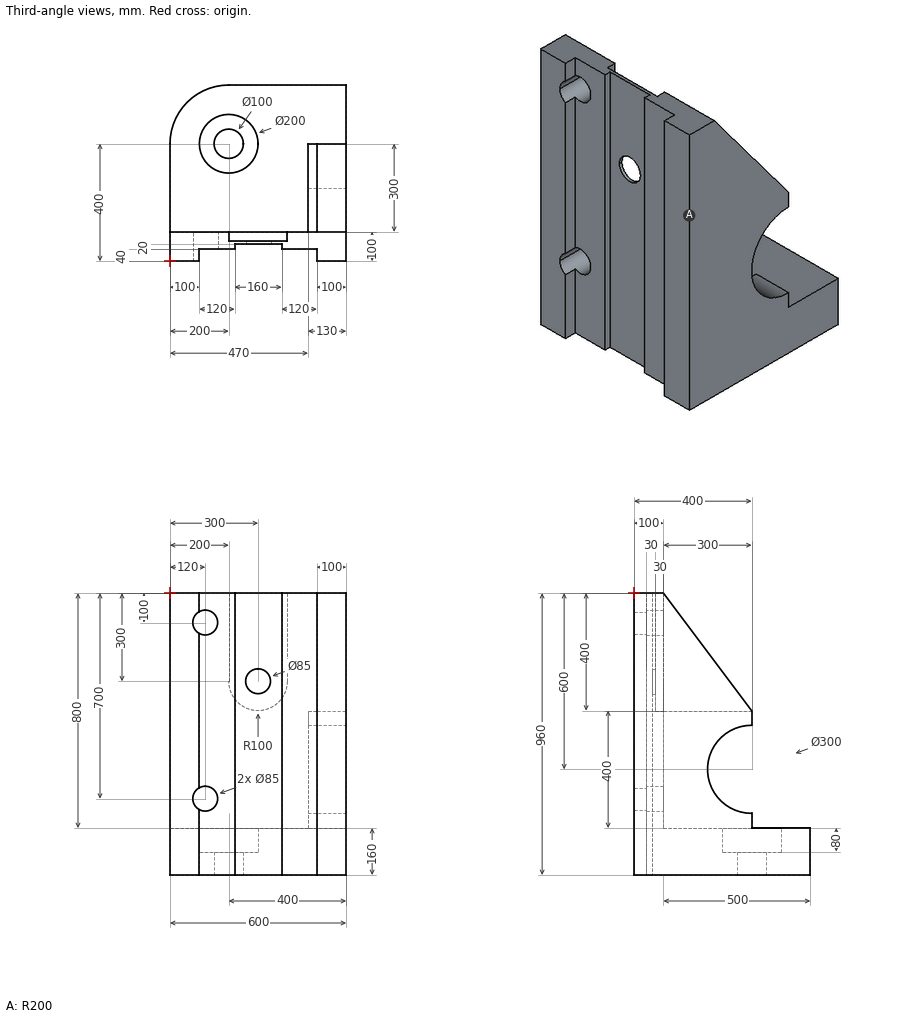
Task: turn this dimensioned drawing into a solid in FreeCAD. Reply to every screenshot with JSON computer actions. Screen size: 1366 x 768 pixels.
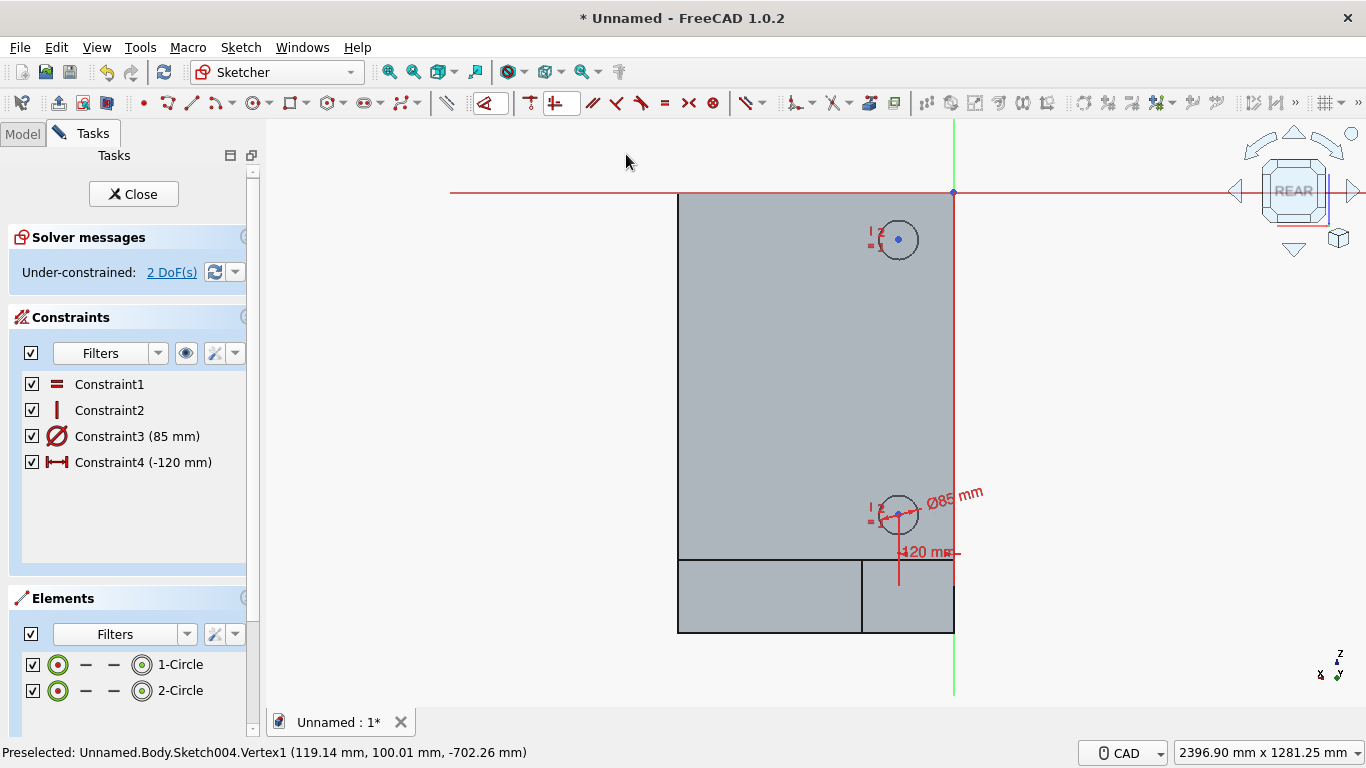
{"action": "left_click", "coordinate": [899, 515]}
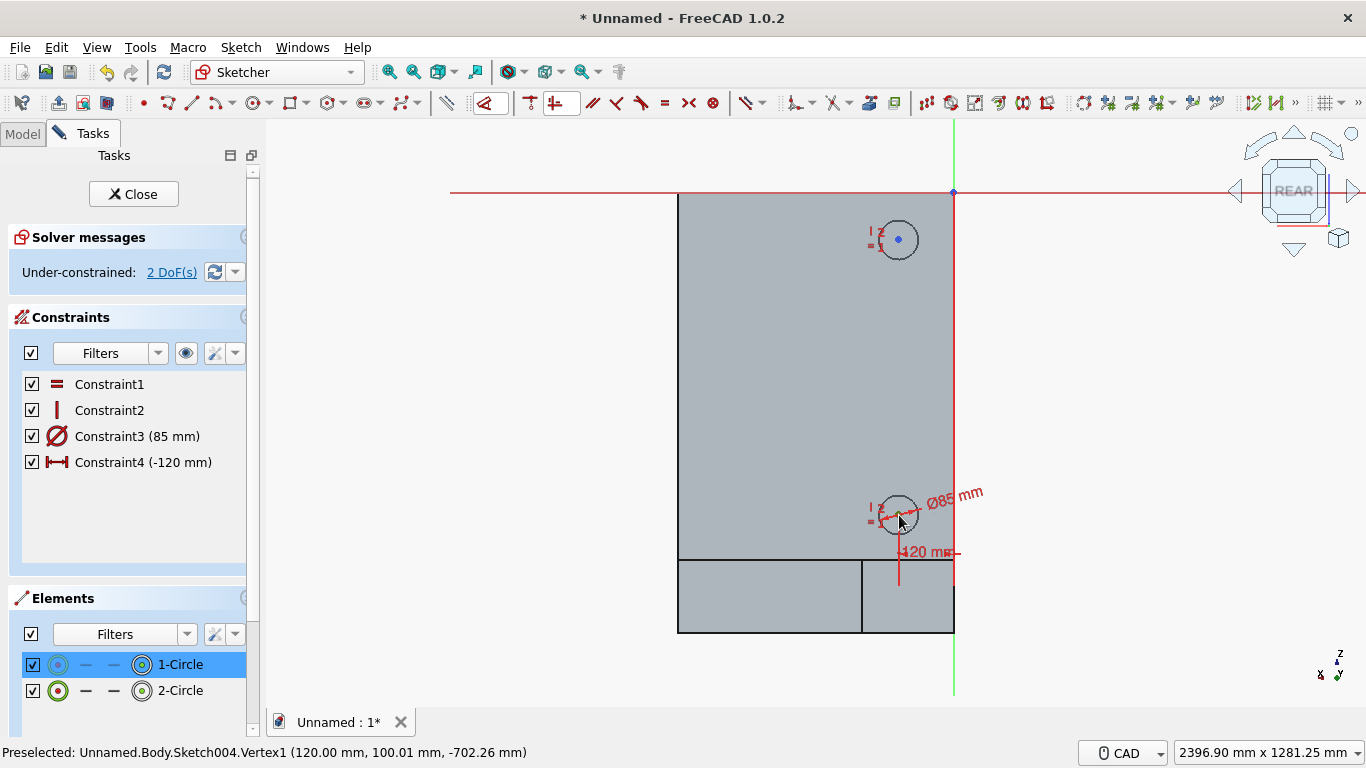
{"action": "left_click", "coordinate": [502, 104]}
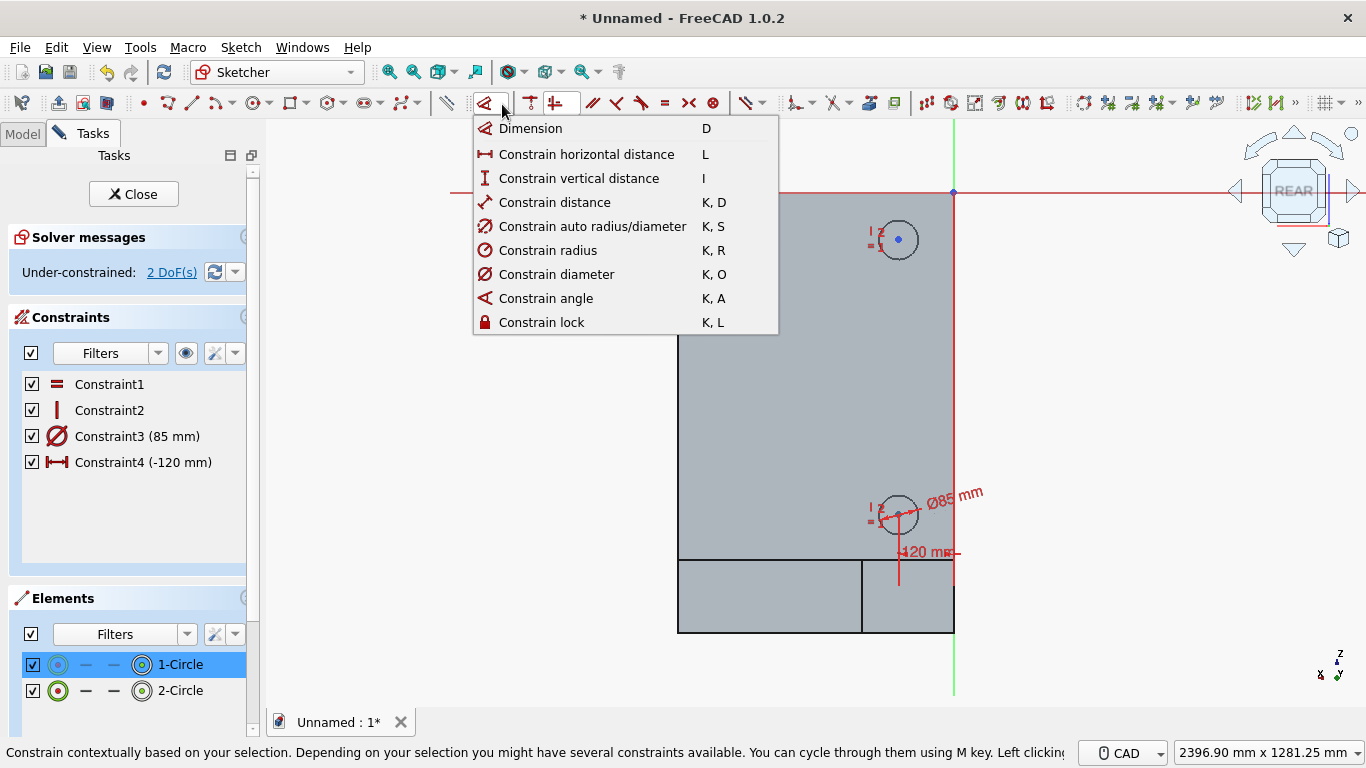
{"action": "left_click", "coordinate": [626, 178]}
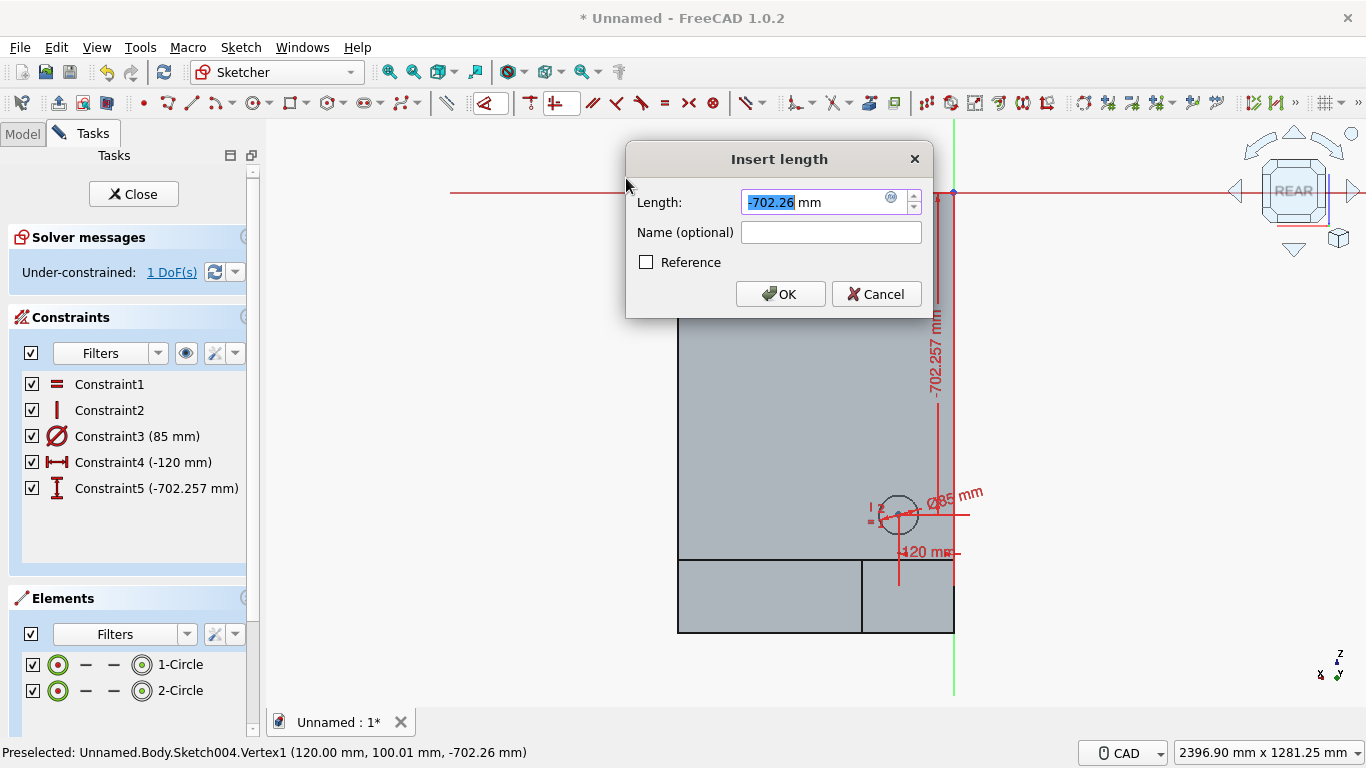
{"action": "type", "text": "-700"}
{"action": "key", "text": "Return"}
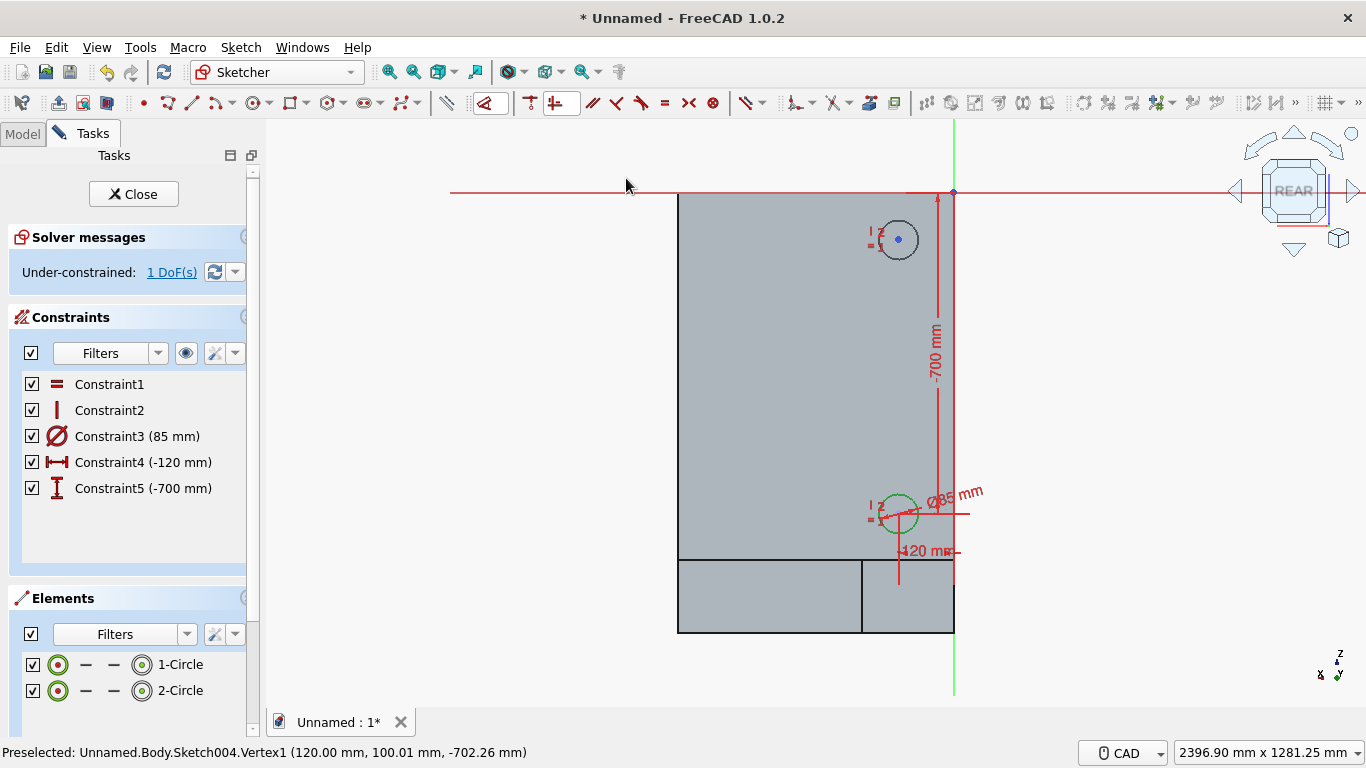
{"action": "left_click", "coordinate": [899, 240]}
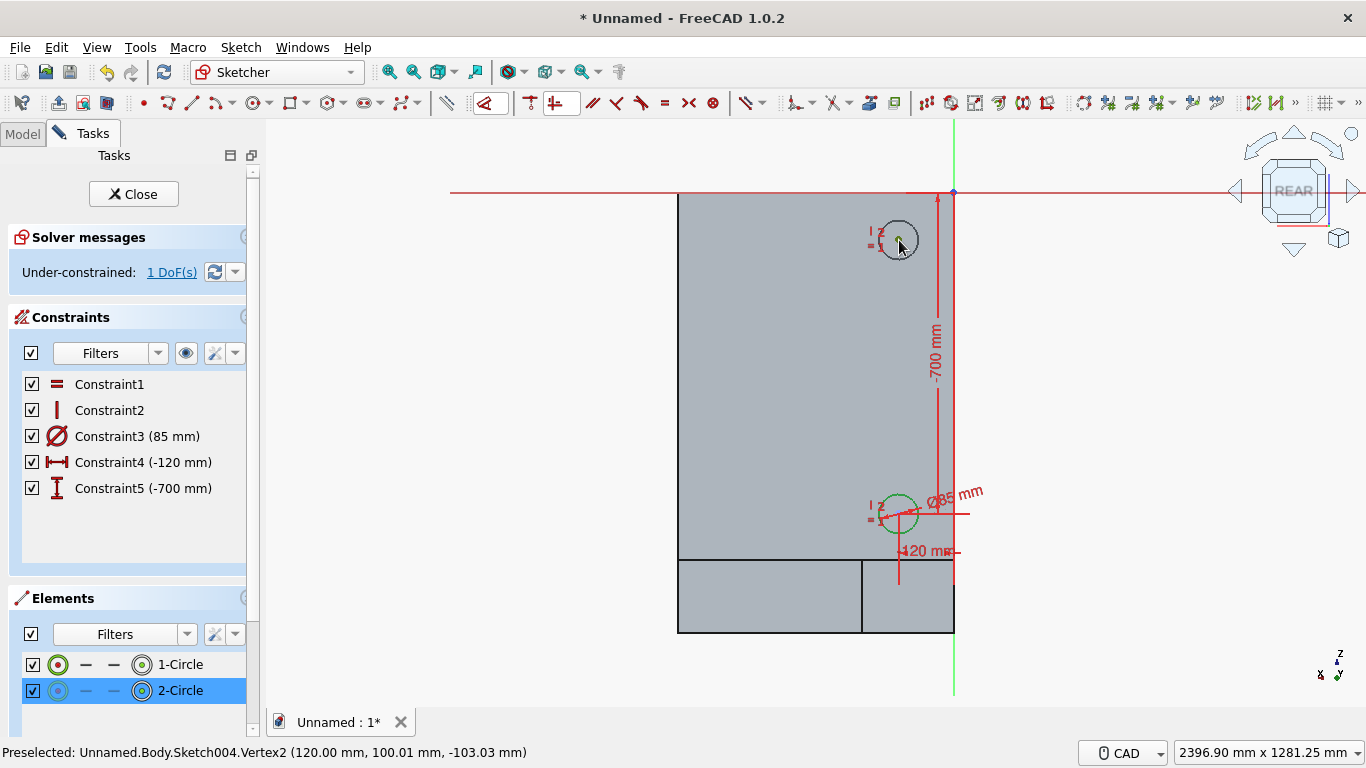
{"action": "key", "text": "i"}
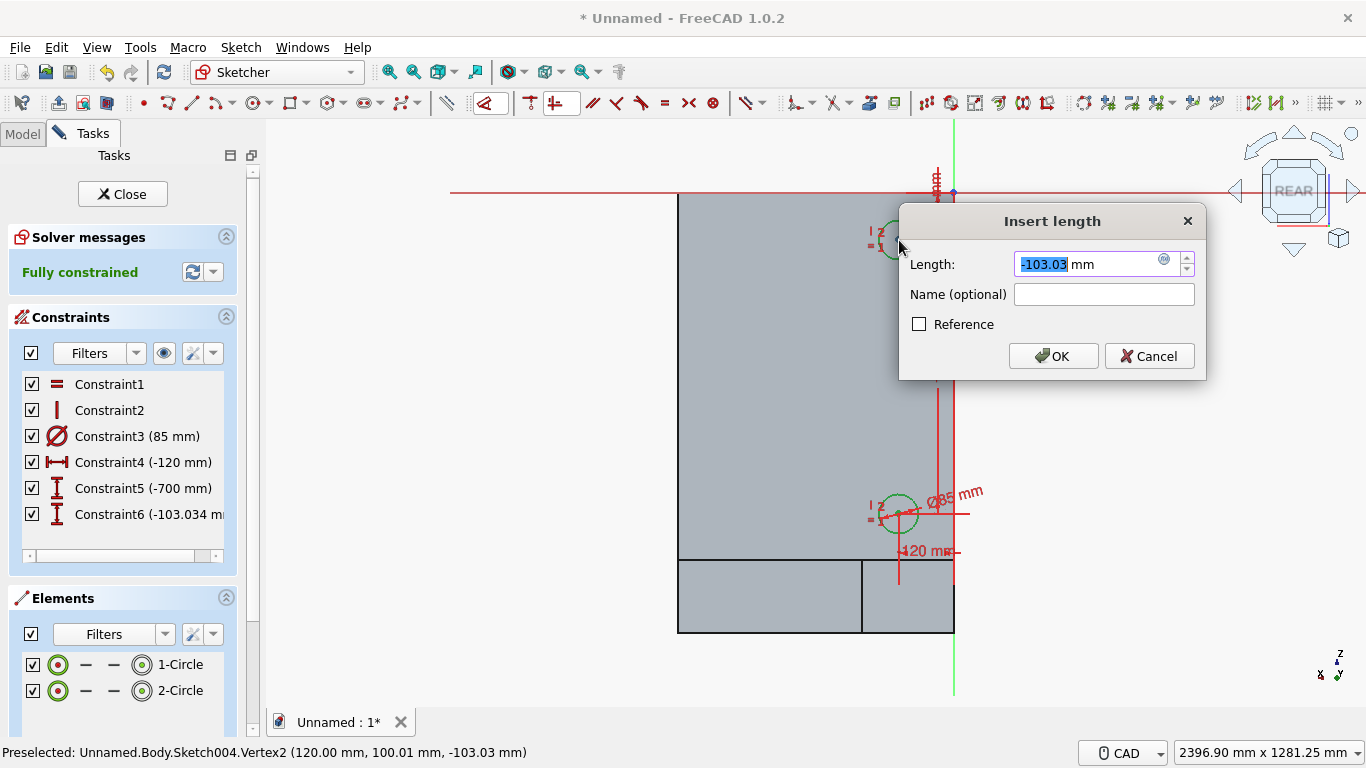
{"action": "type", "text": "-100"}
{"action": "key", "text": "Return"}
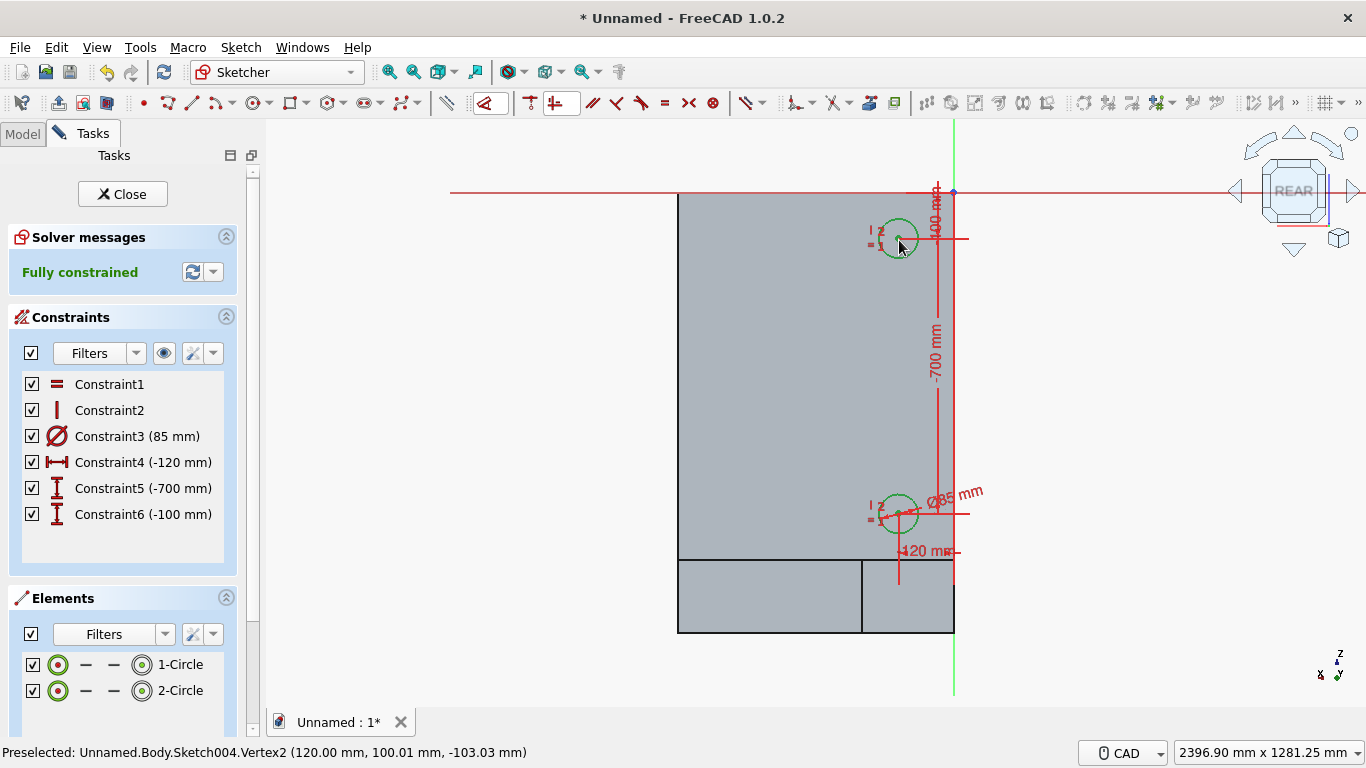
{"action": "left_click", "coordinate": [123, 194]}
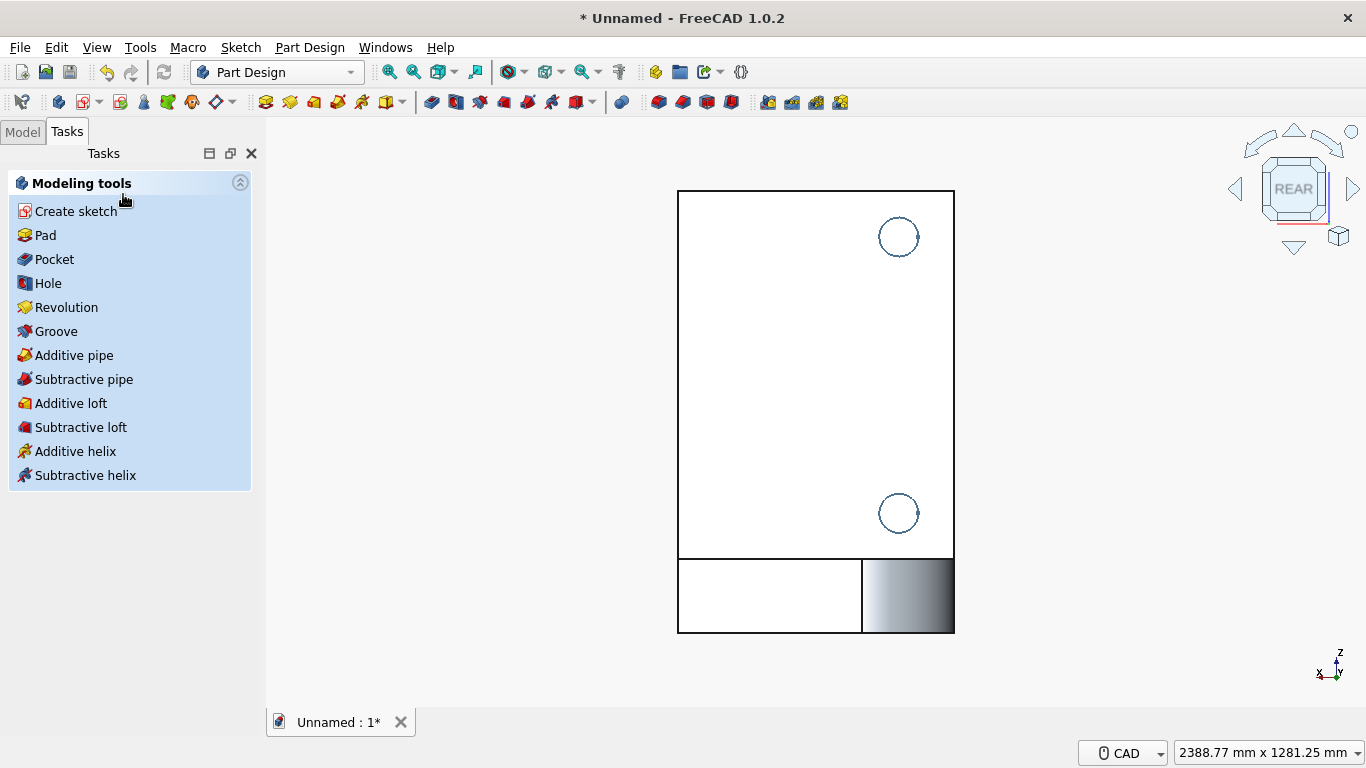
{"action": "left_click", "coordinate": [432, 102]}